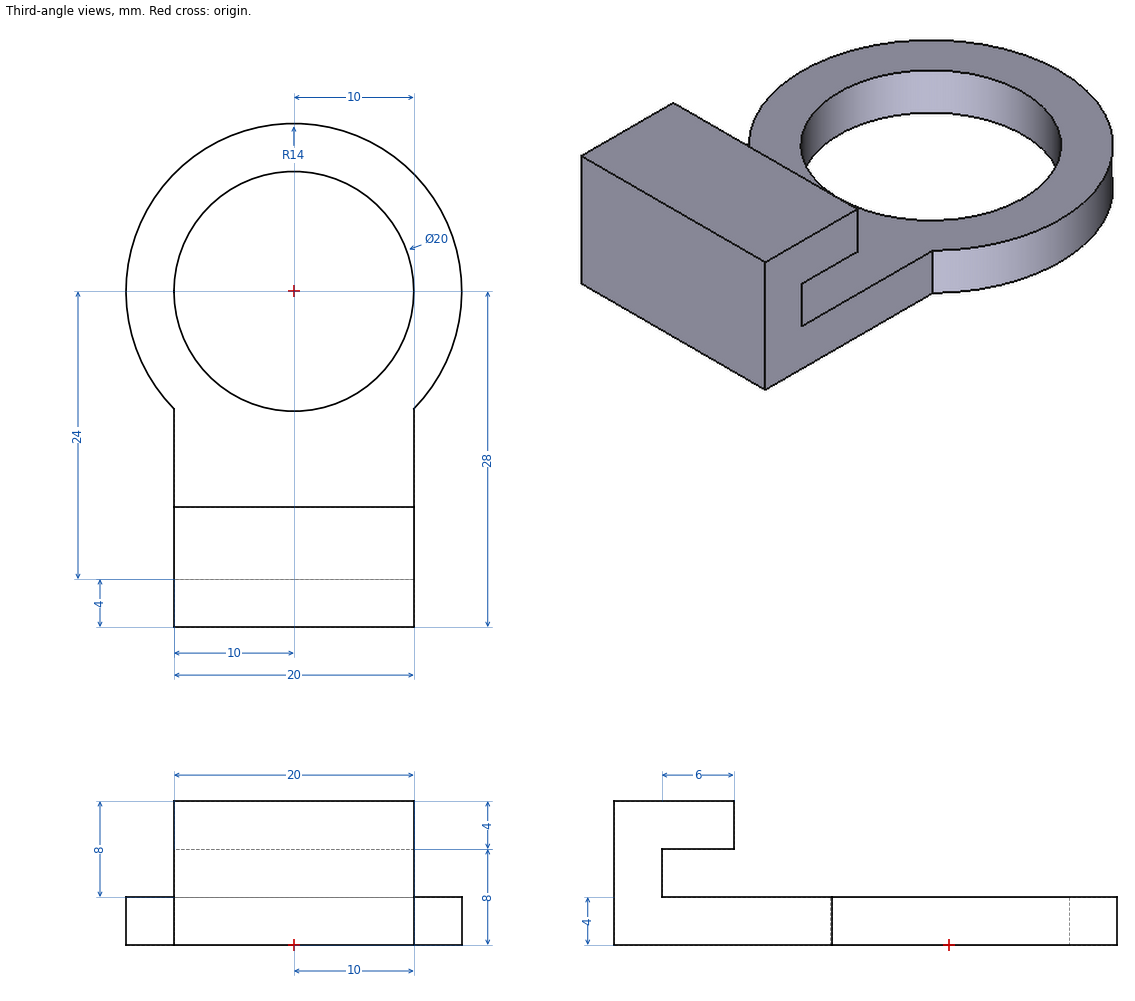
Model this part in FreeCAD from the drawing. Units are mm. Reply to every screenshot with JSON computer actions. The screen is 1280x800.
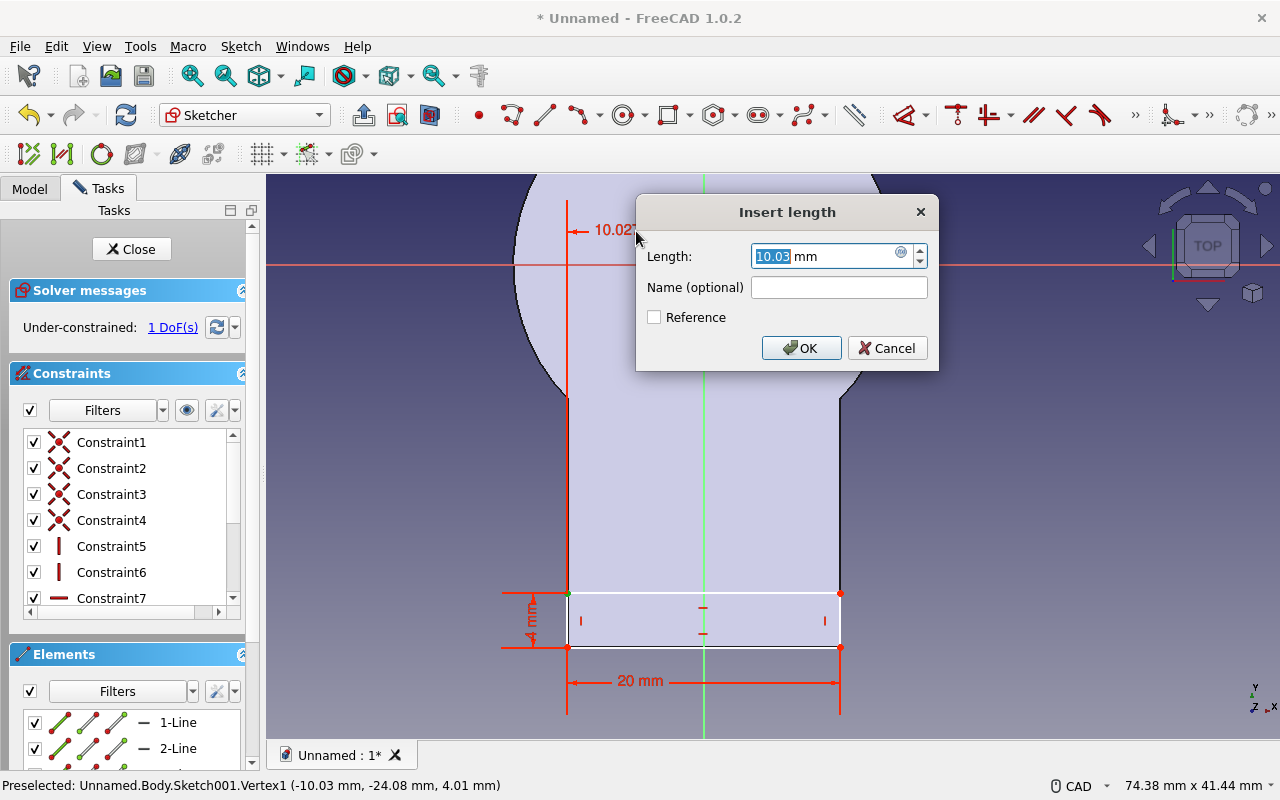
{"action": "type", "text": "10"}
{"action": "key", "text": "Return"}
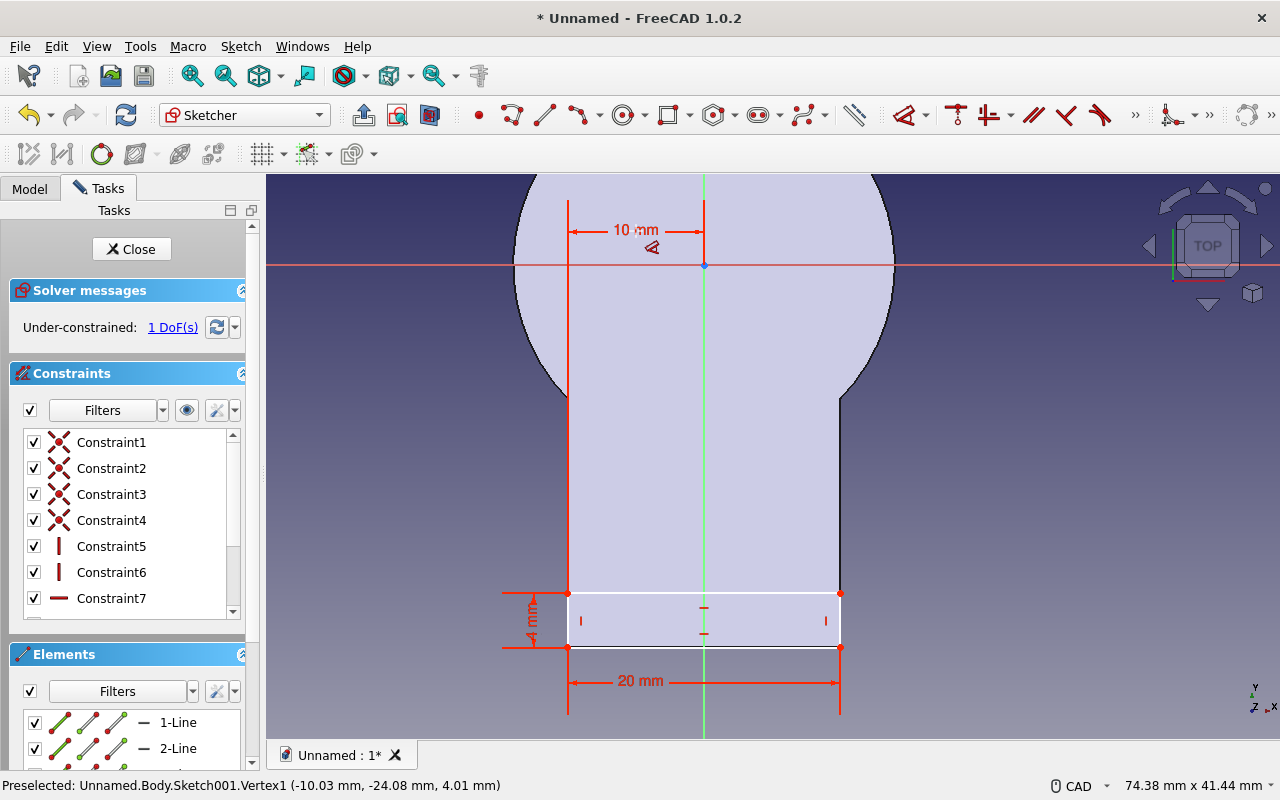
{"action": "left_click", "coordinate": [568, 593]}
{"action": "left_click", "coordinate": [534, 429]}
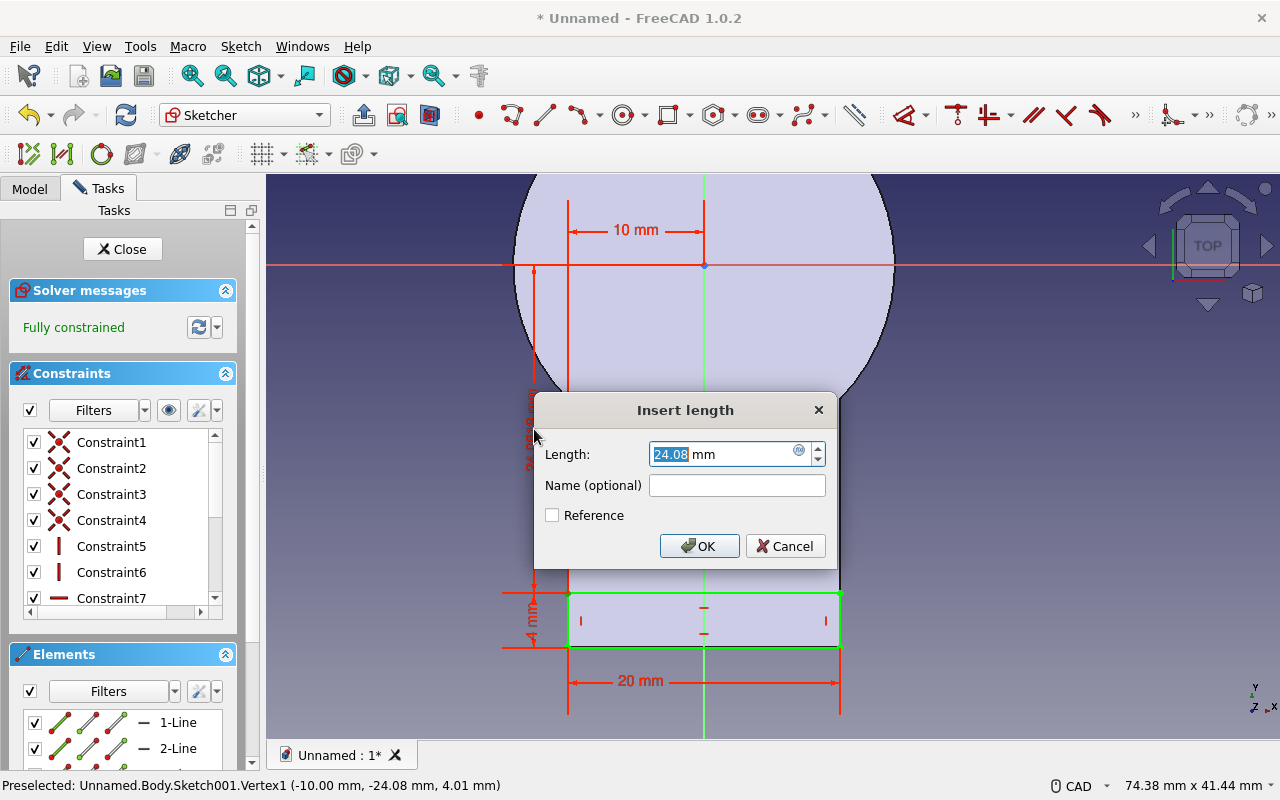
{"action": "type", "text": "24"}
{"action": "key", "text": "Return"}
{"action": "key", "text": "Escape"}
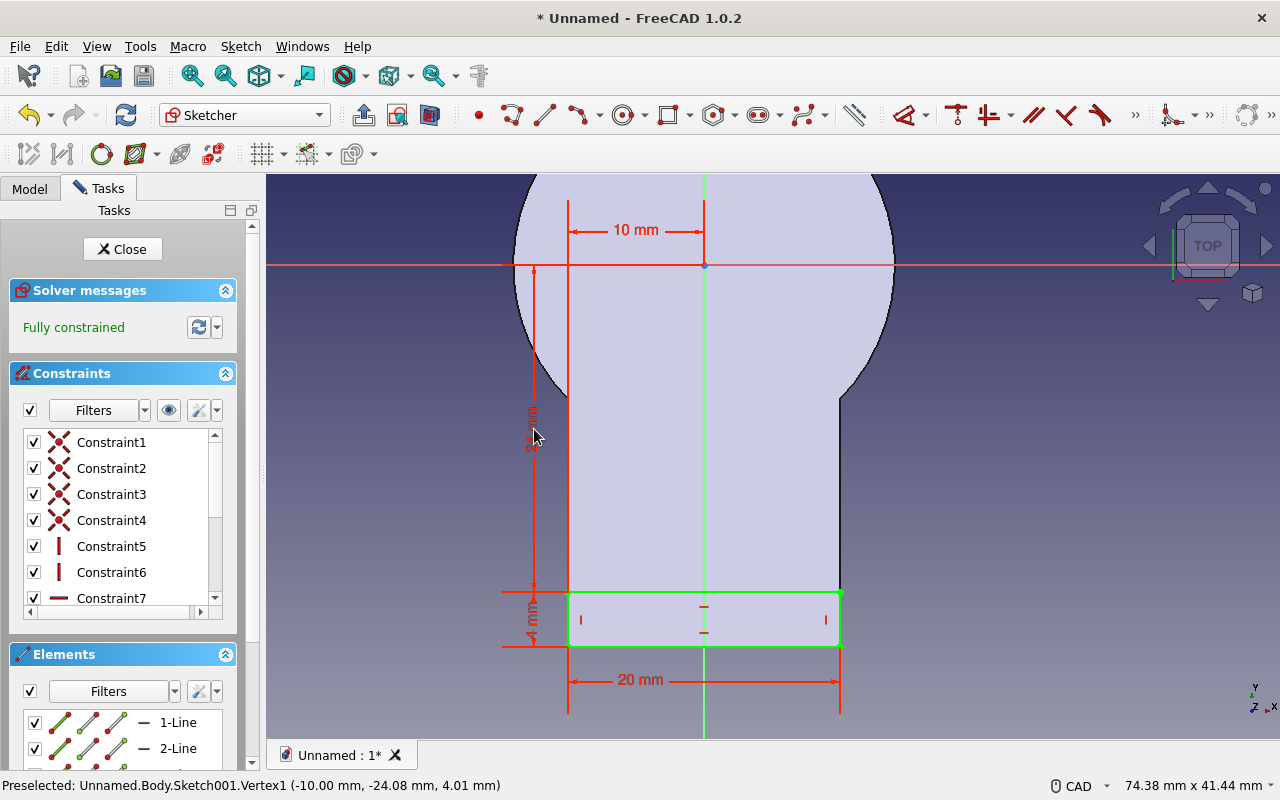
{"action": "left_click", "coordinate": [123, 249]}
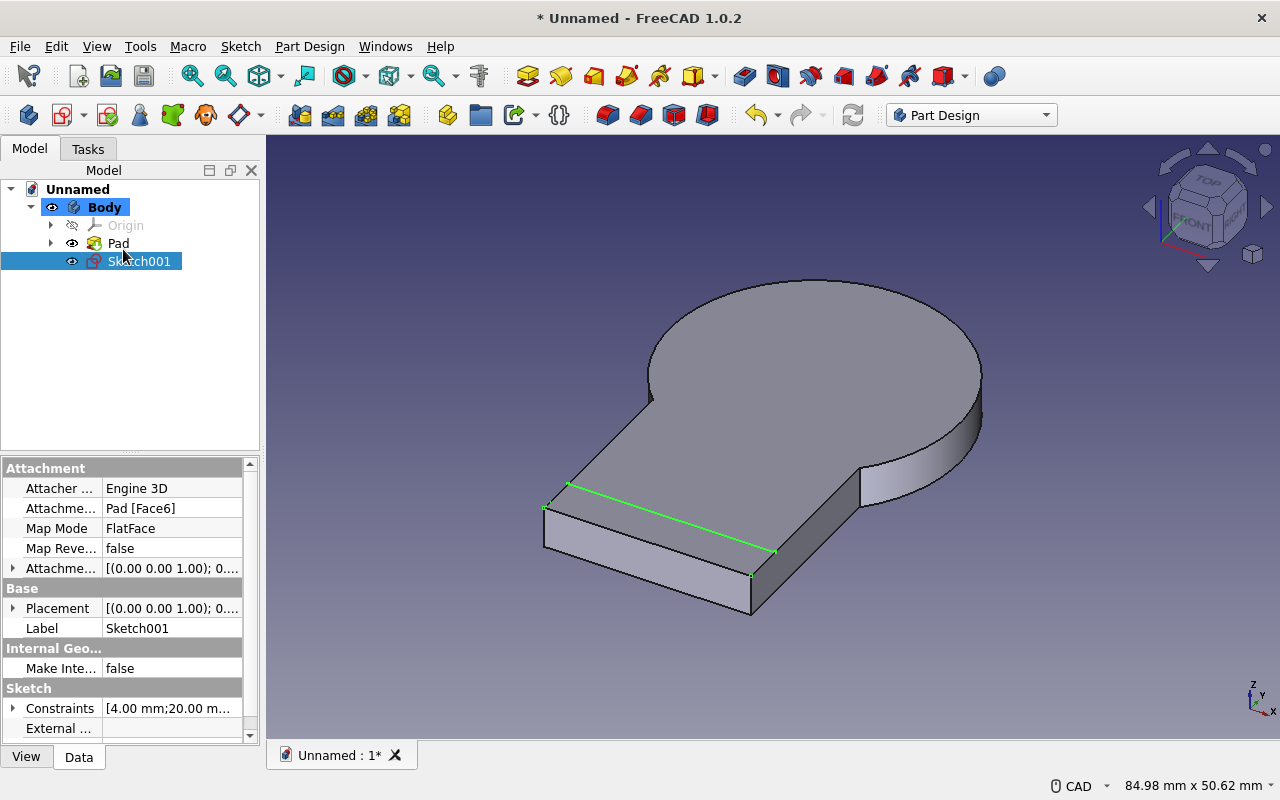
{"action": "left_click", "coordinate": [528, 76]}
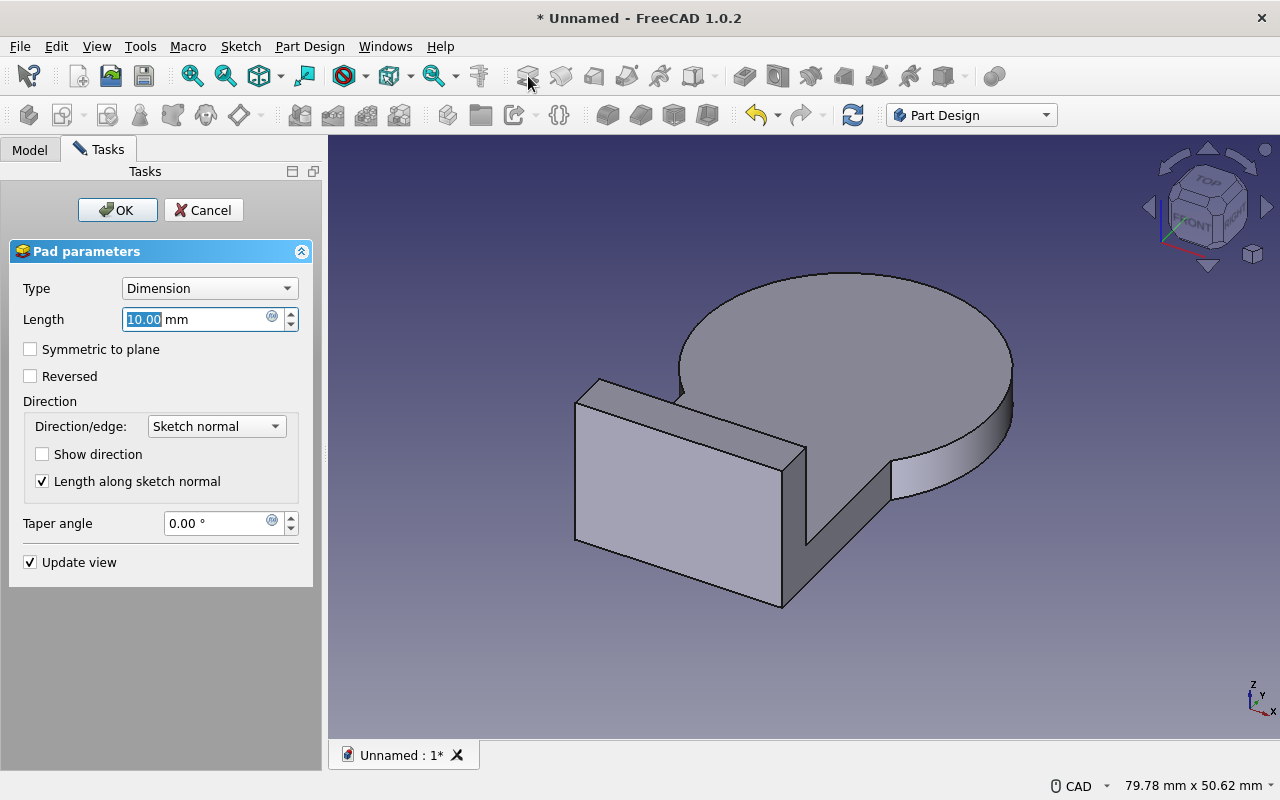
{"action": "type", "text": "8"}
{"action": "key", "text": "Tab"}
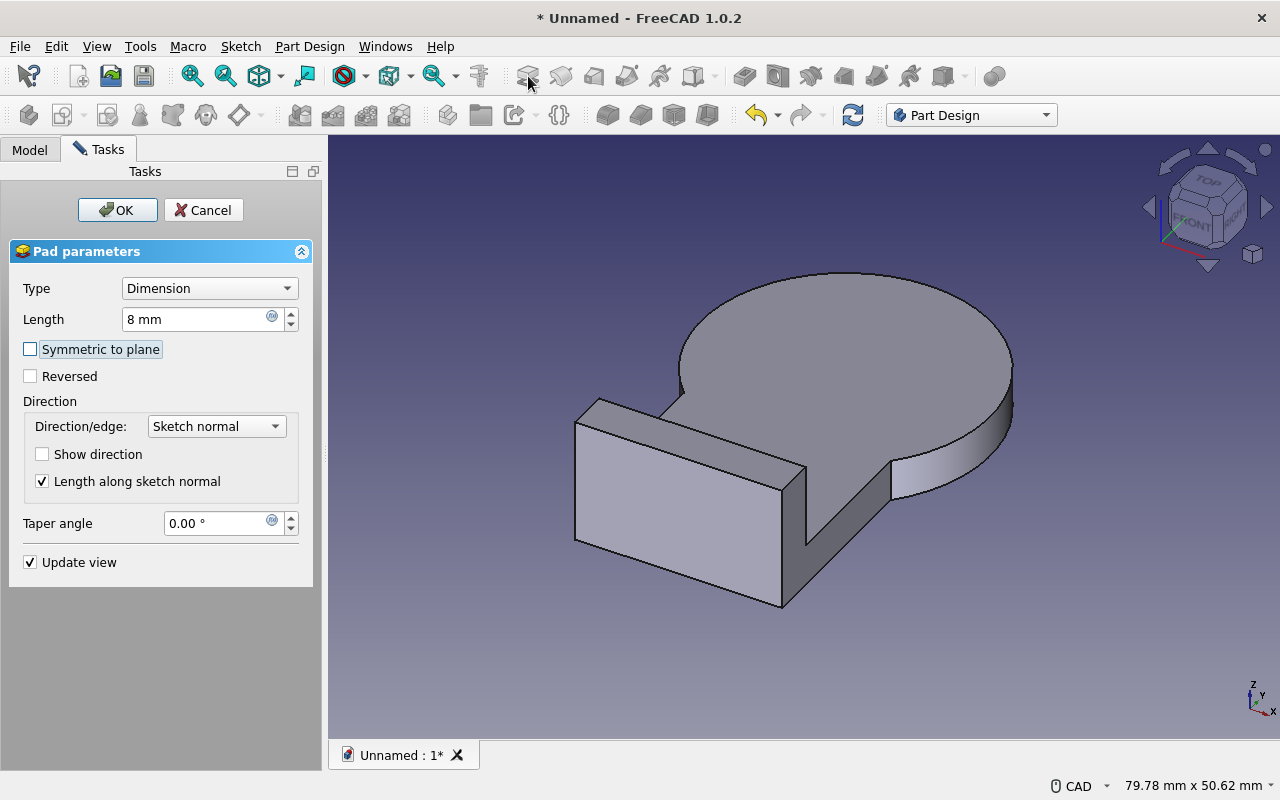
{"action": "left_click", "coordinate": [118, 210]}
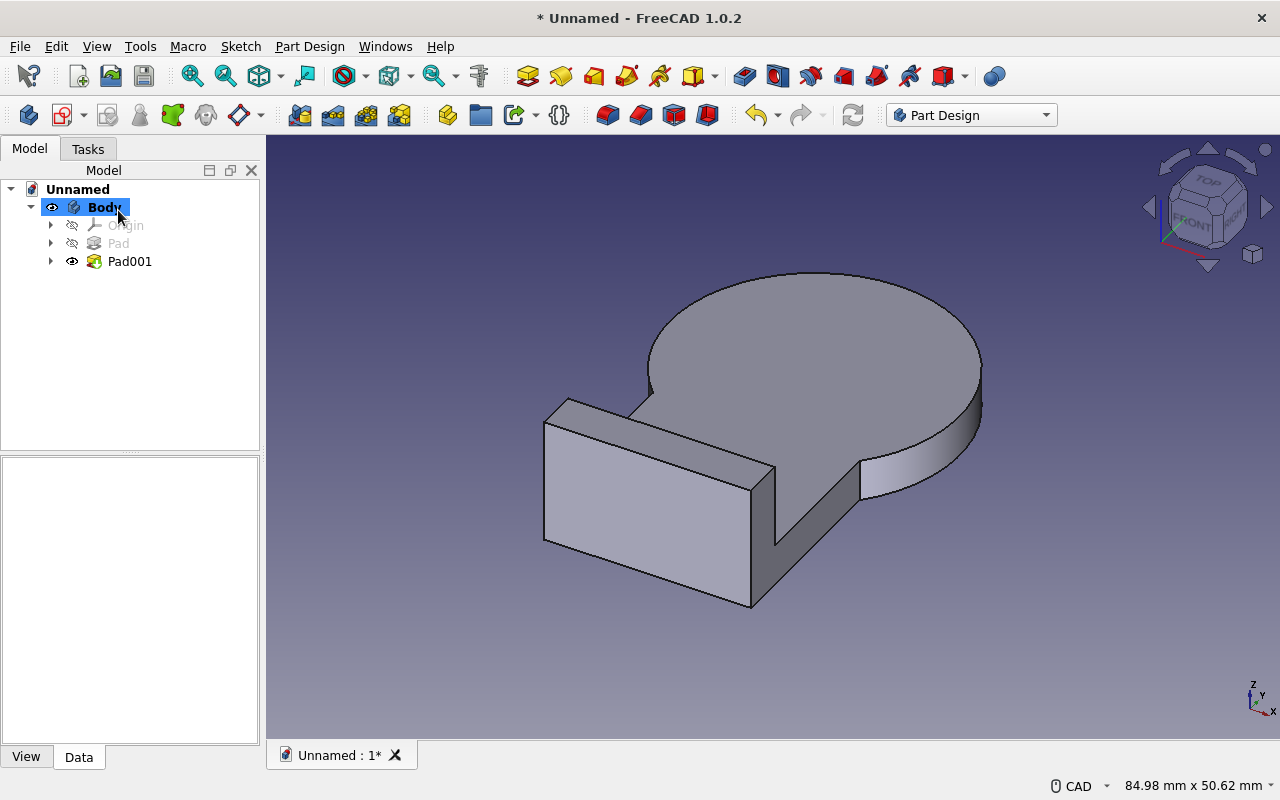
{"action": "key", "text": "4"}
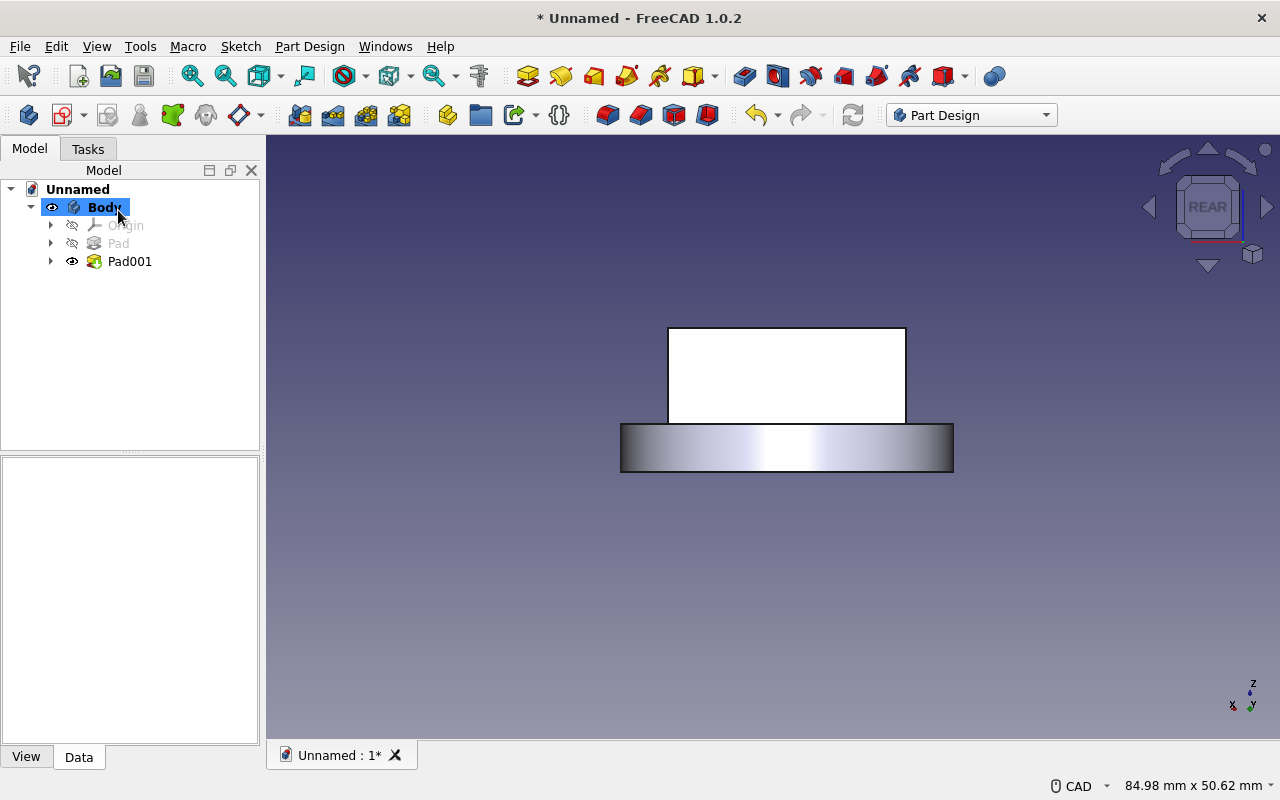
{"action": "left_click", "coordinate": [193, 76]}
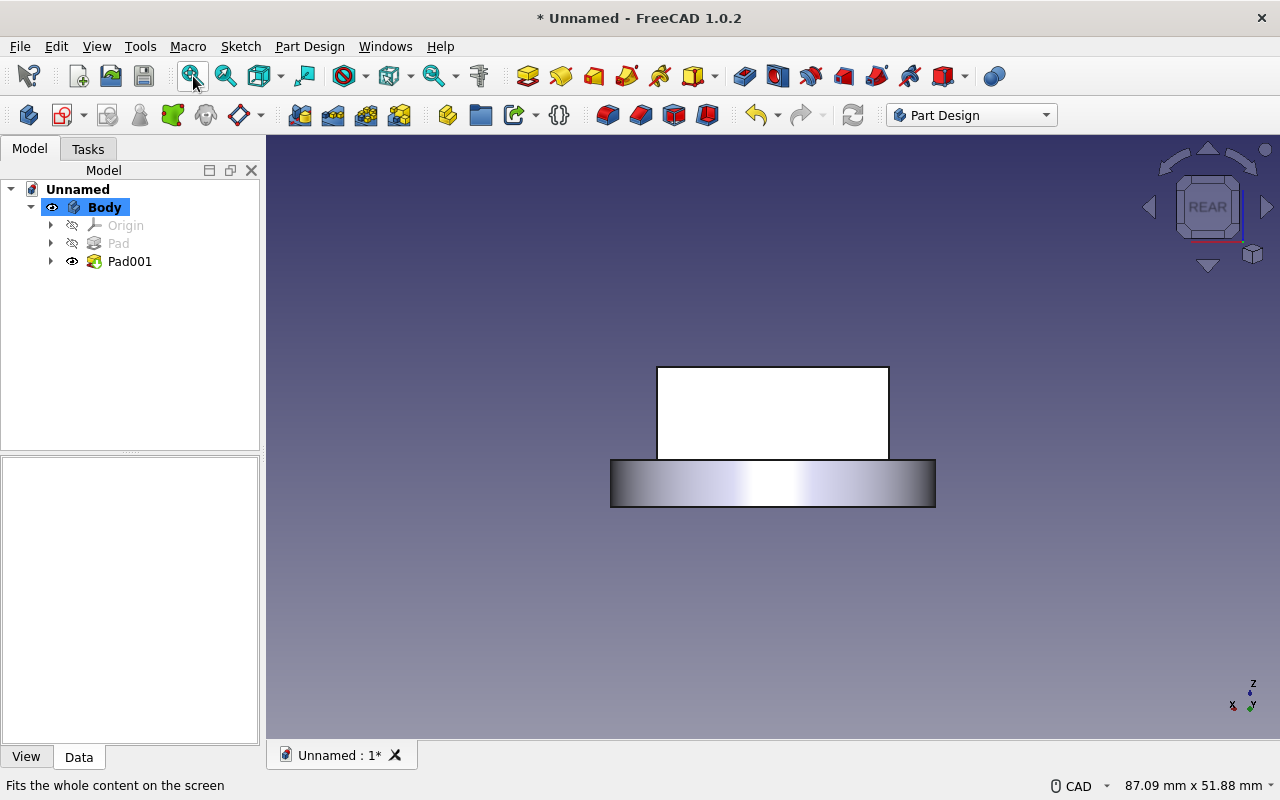
{"action": "left_click", "coordinate": [706, 413]}